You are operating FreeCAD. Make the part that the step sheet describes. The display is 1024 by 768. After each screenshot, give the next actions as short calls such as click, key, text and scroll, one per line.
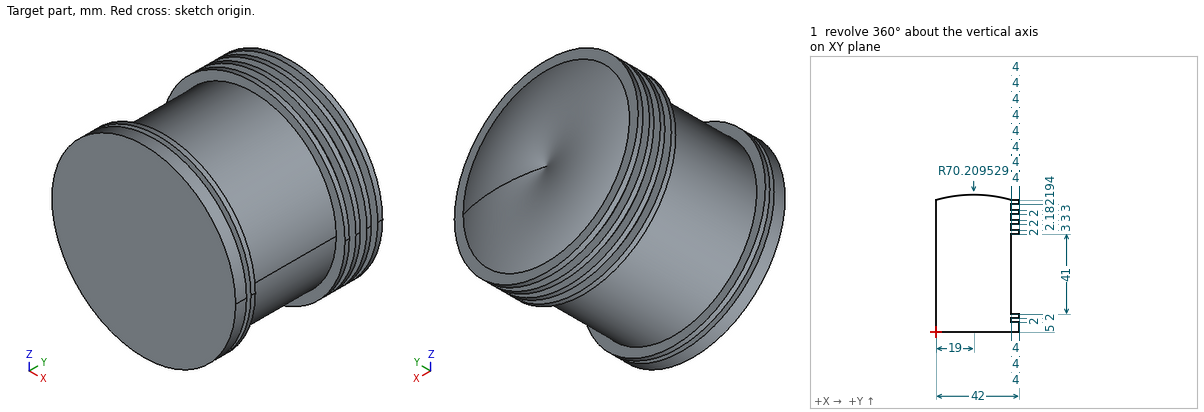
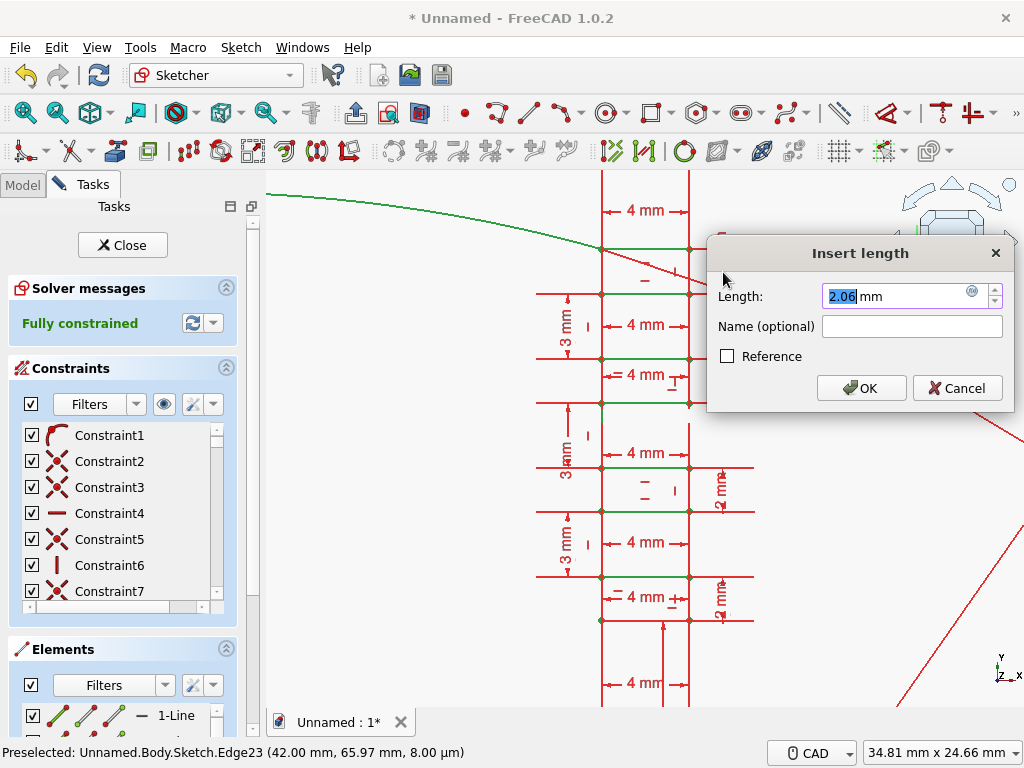
text(2.182194)
key(Return)
key(Escape)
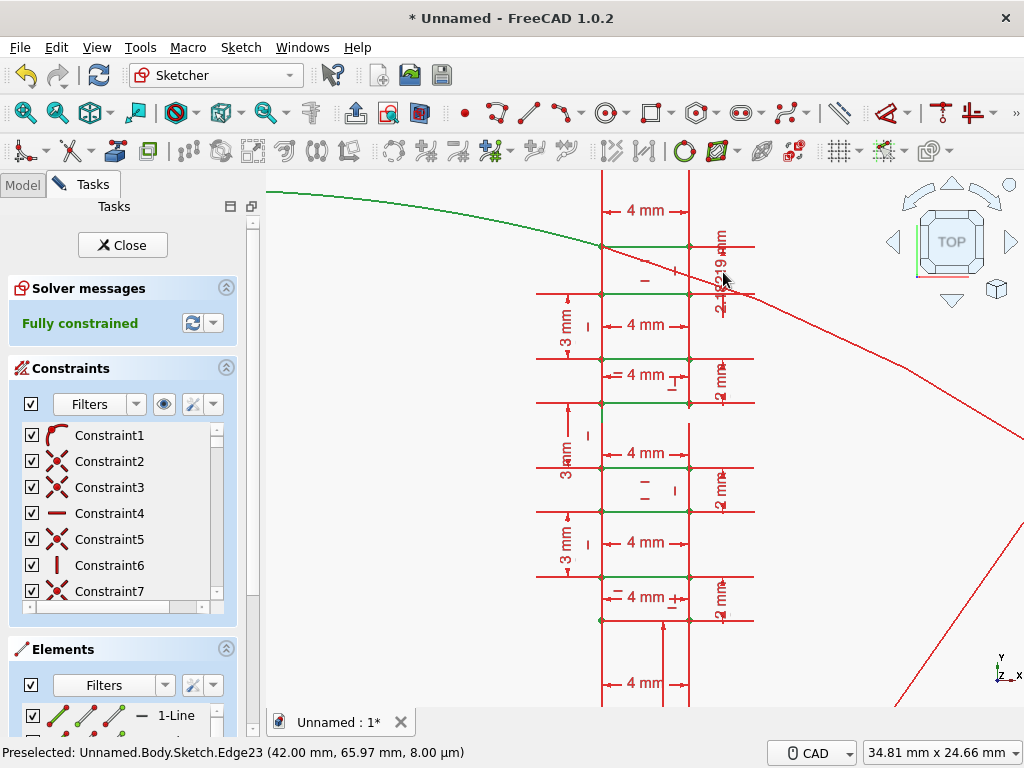
click(123, 245)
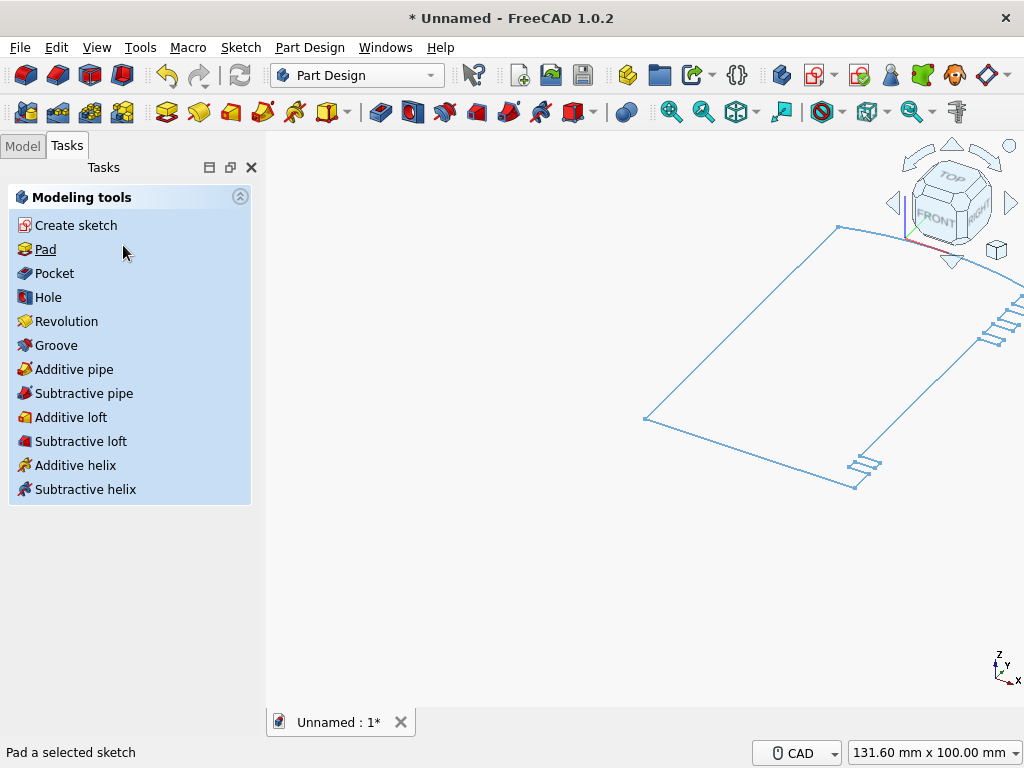
click(200, 112)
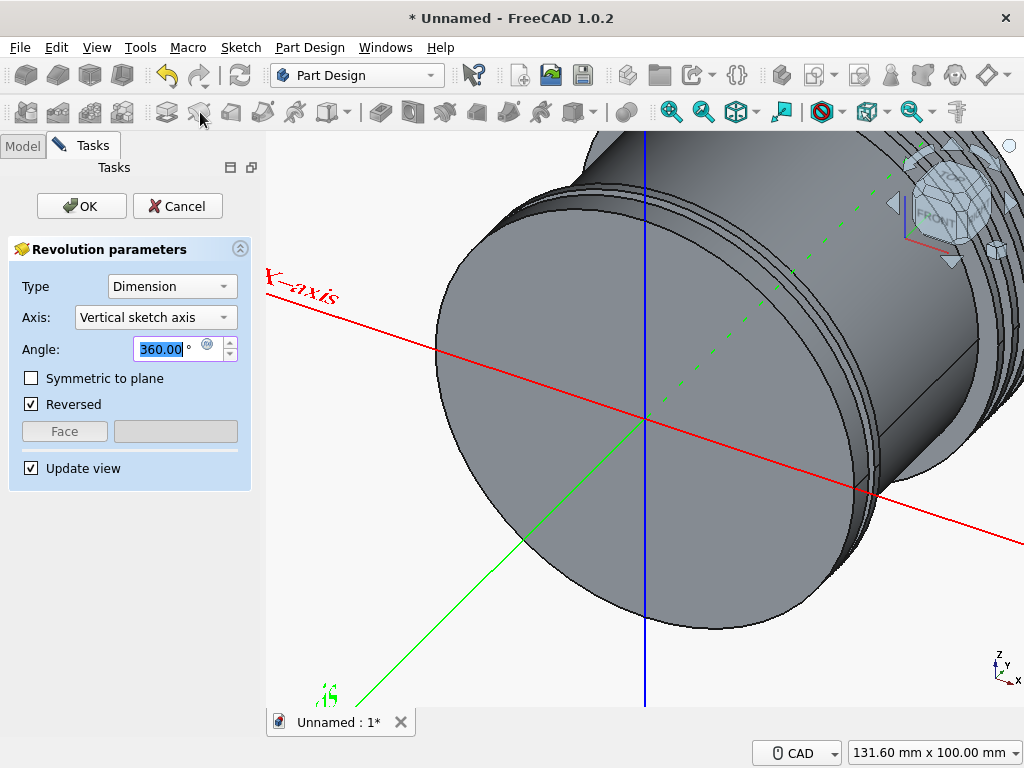
click(82, 206)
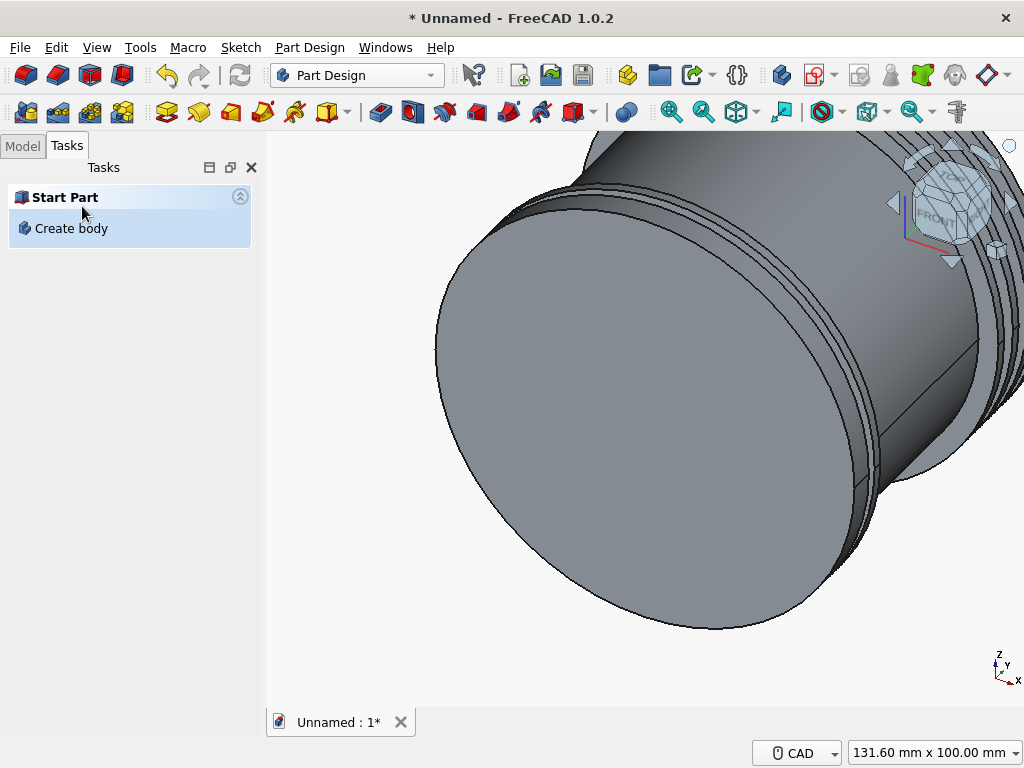
key(0)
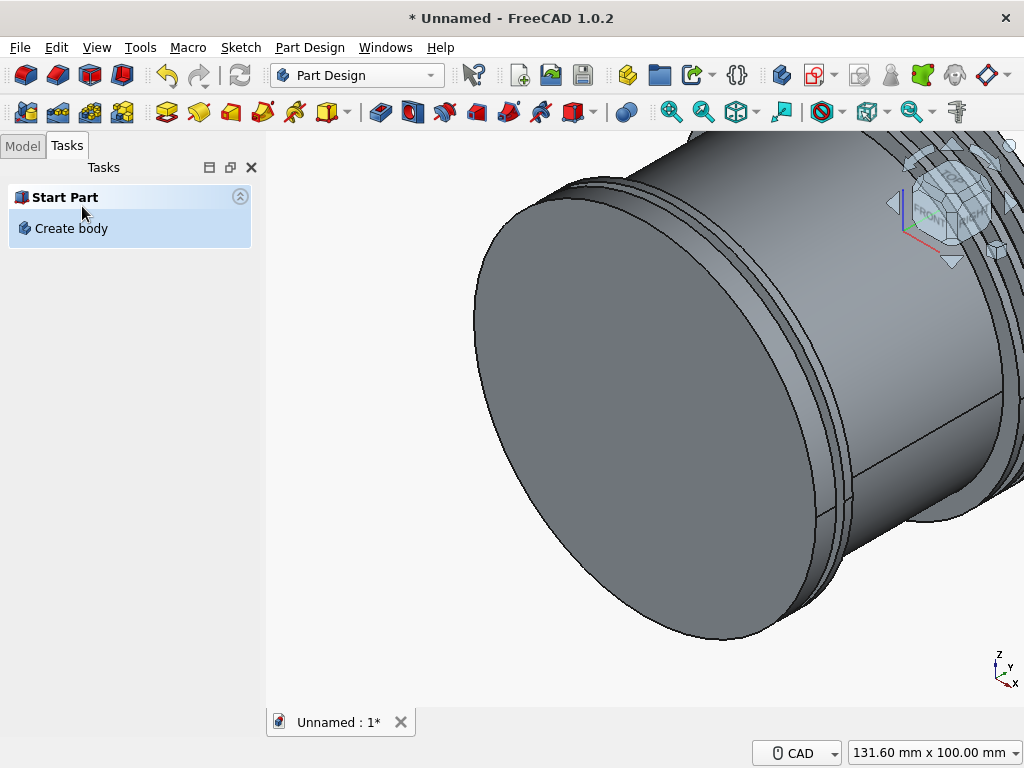
key(v)
key(f)